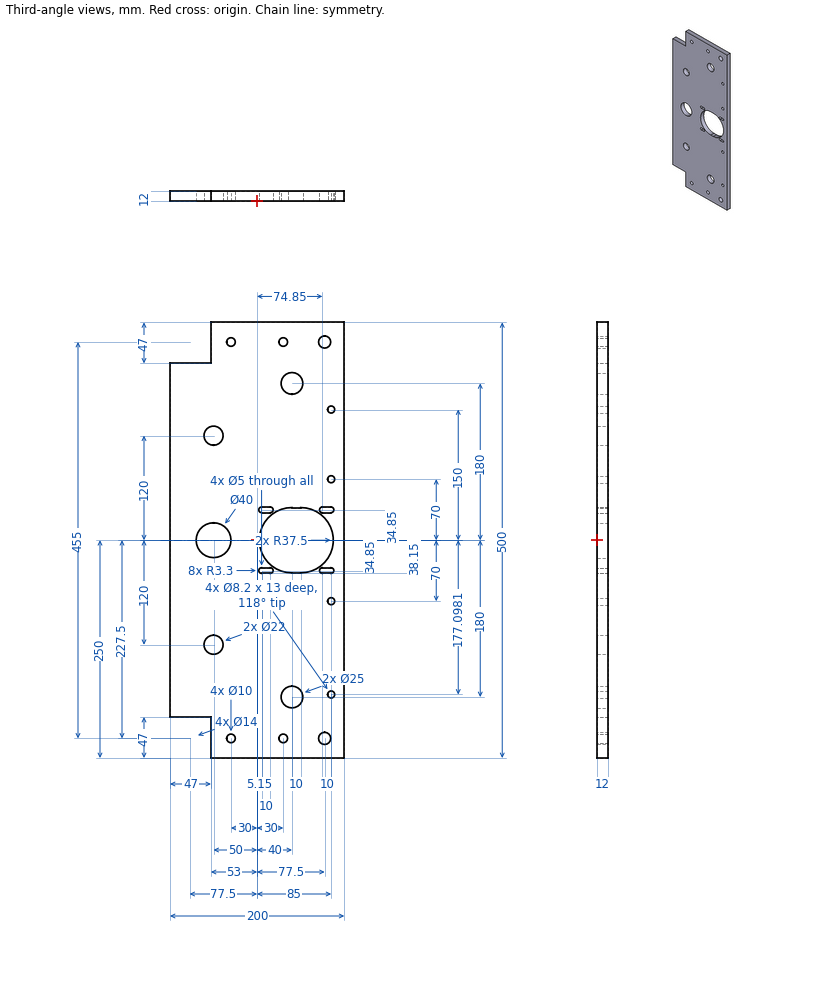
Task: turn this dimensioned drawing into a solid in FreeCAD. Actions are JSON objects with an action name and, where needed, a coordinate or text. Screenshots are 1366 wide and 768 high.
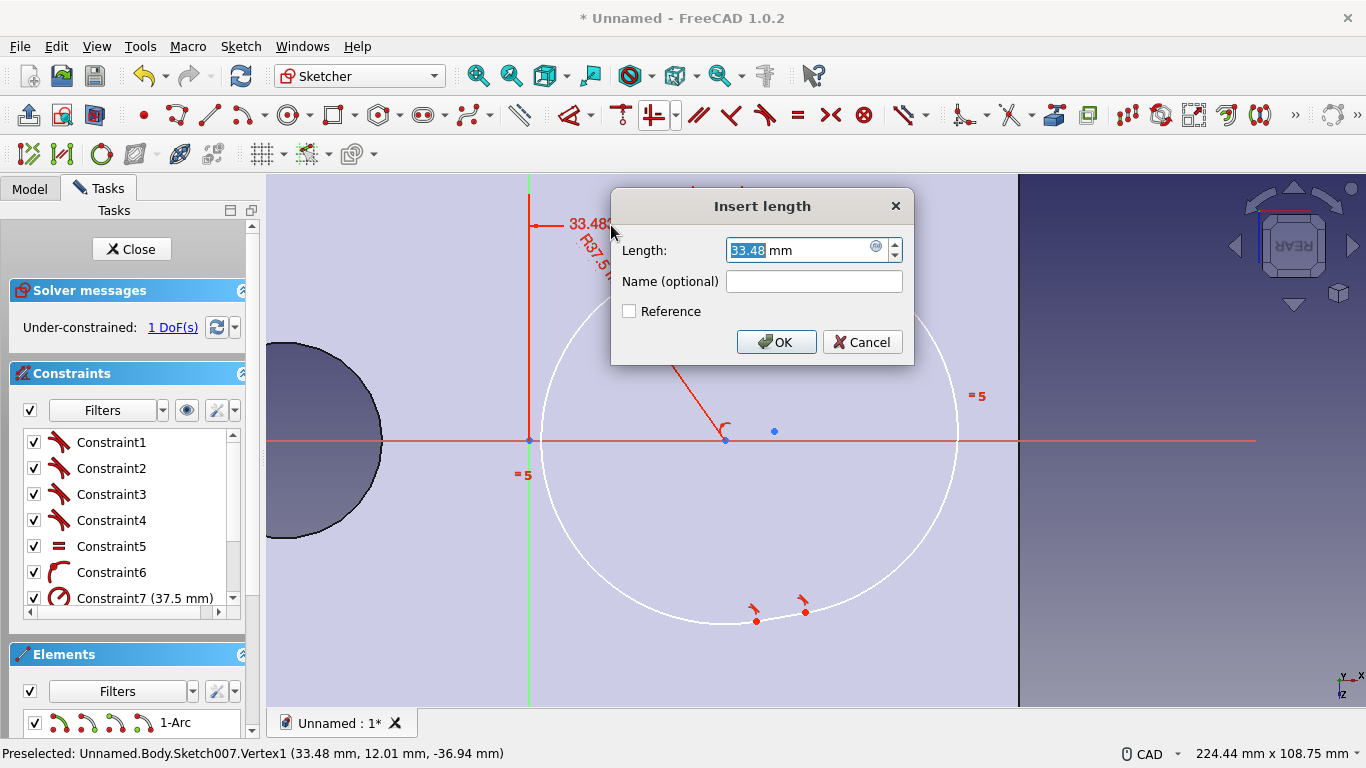
{"action": "type", "text": "40"}
{"action": "key", "text": "Return"}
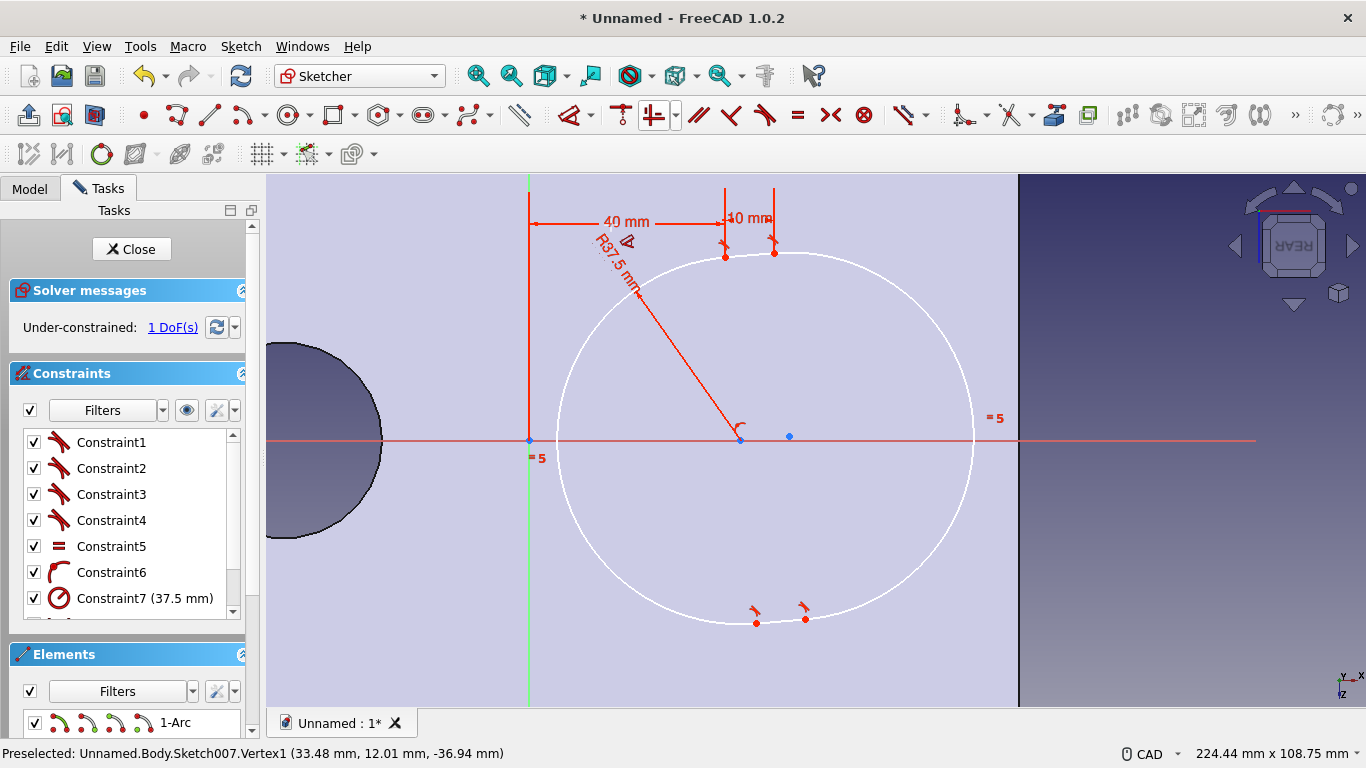
{"action": "left_click", "coordinate": [757, 624]}
{"action": "left_click", "coordinate": [643, 658]}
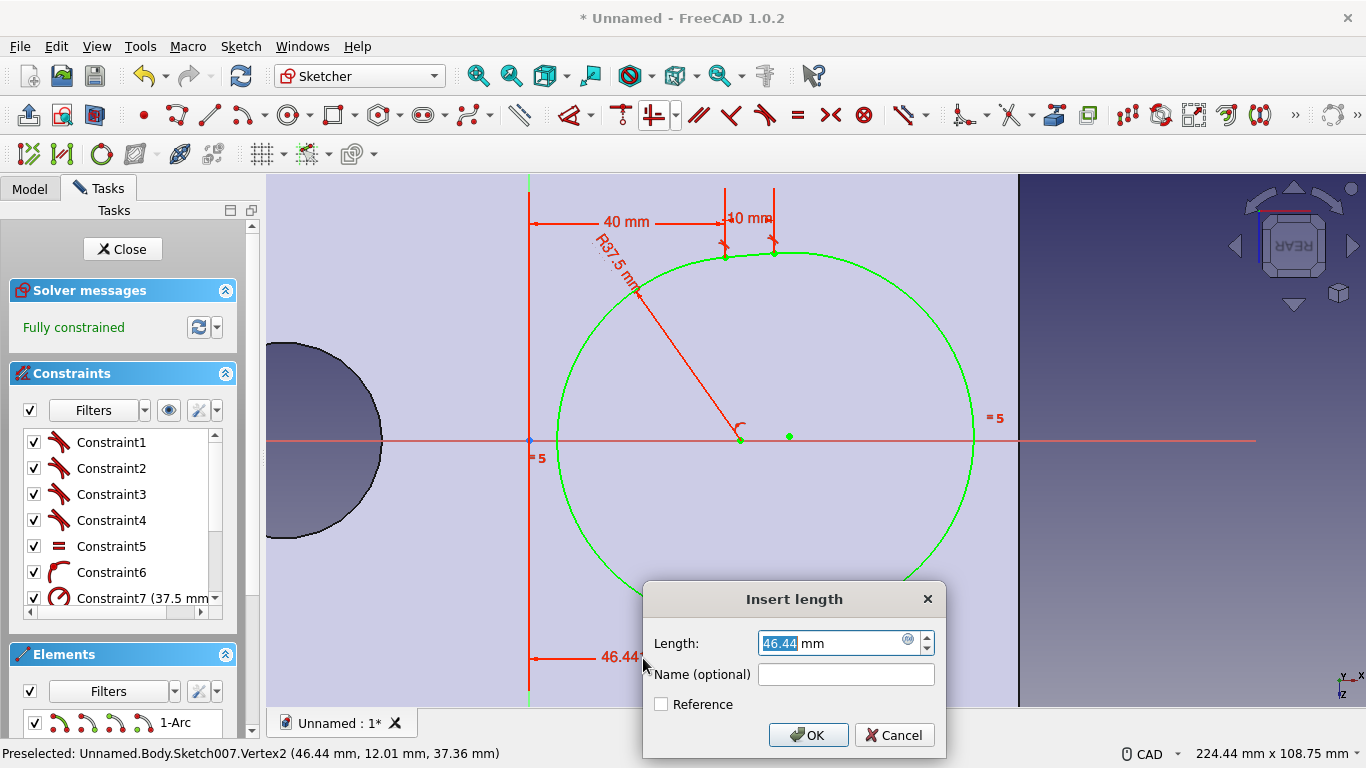
{"action": "type", "text": "40"}
{"action": "key", "text": "Return"}
{"action": "key", "text": "Escape"}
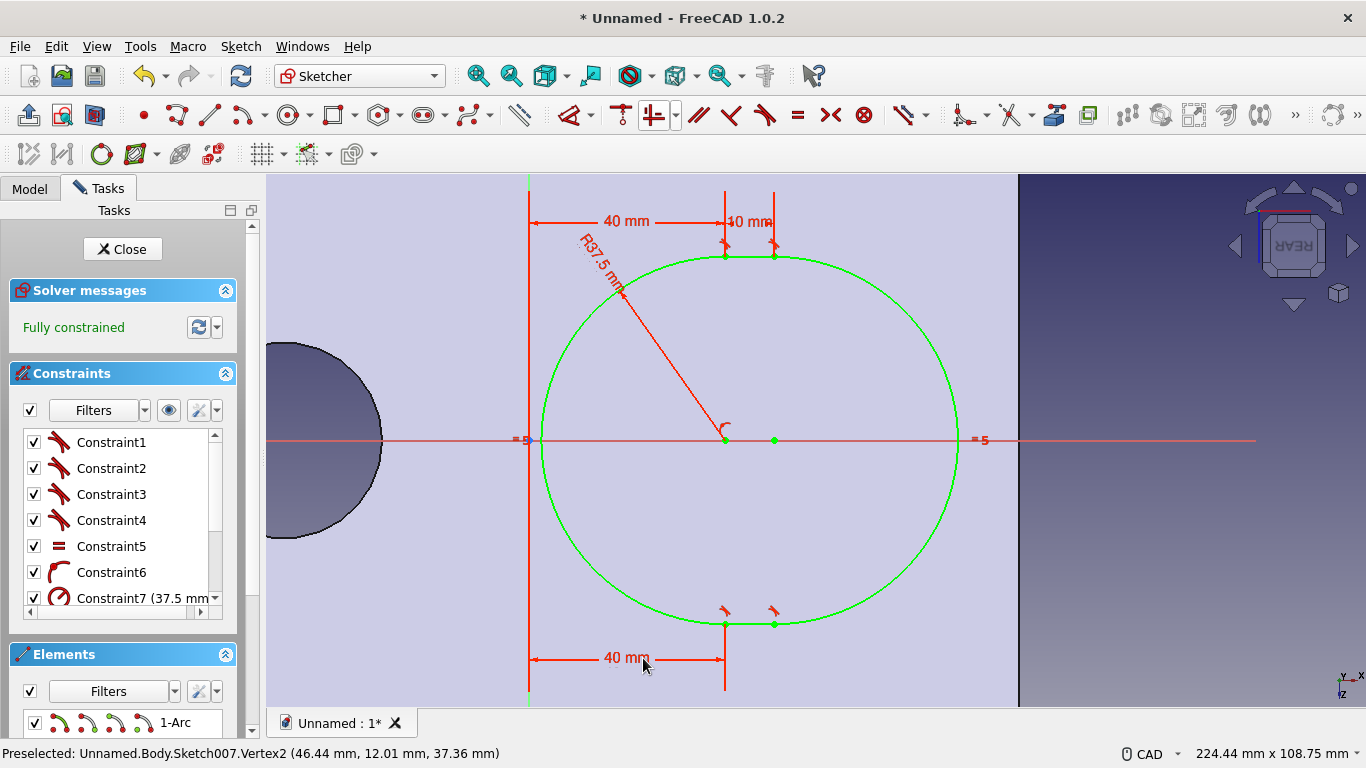
{"action": "left_click", "coordinate": [123, 249]}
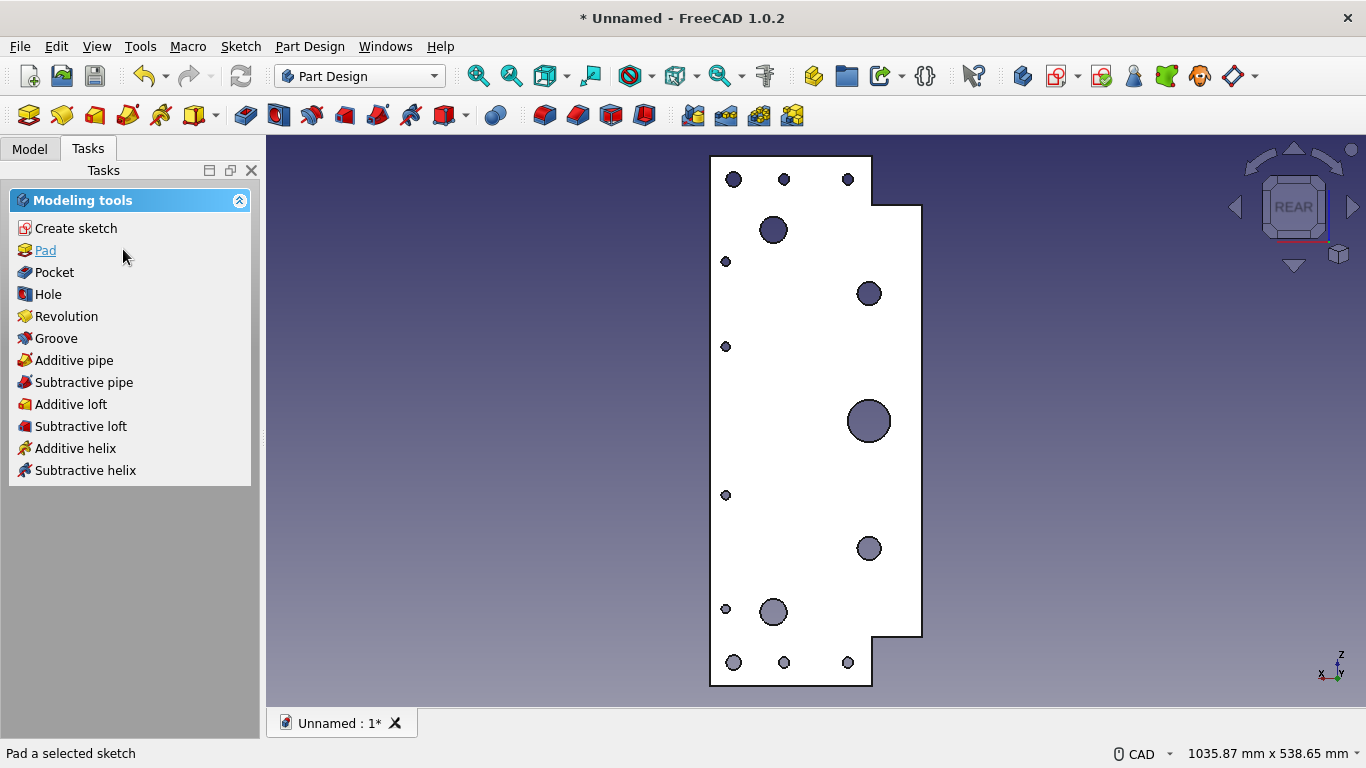
{"action": "left_click", "coordinate": [246, 116]}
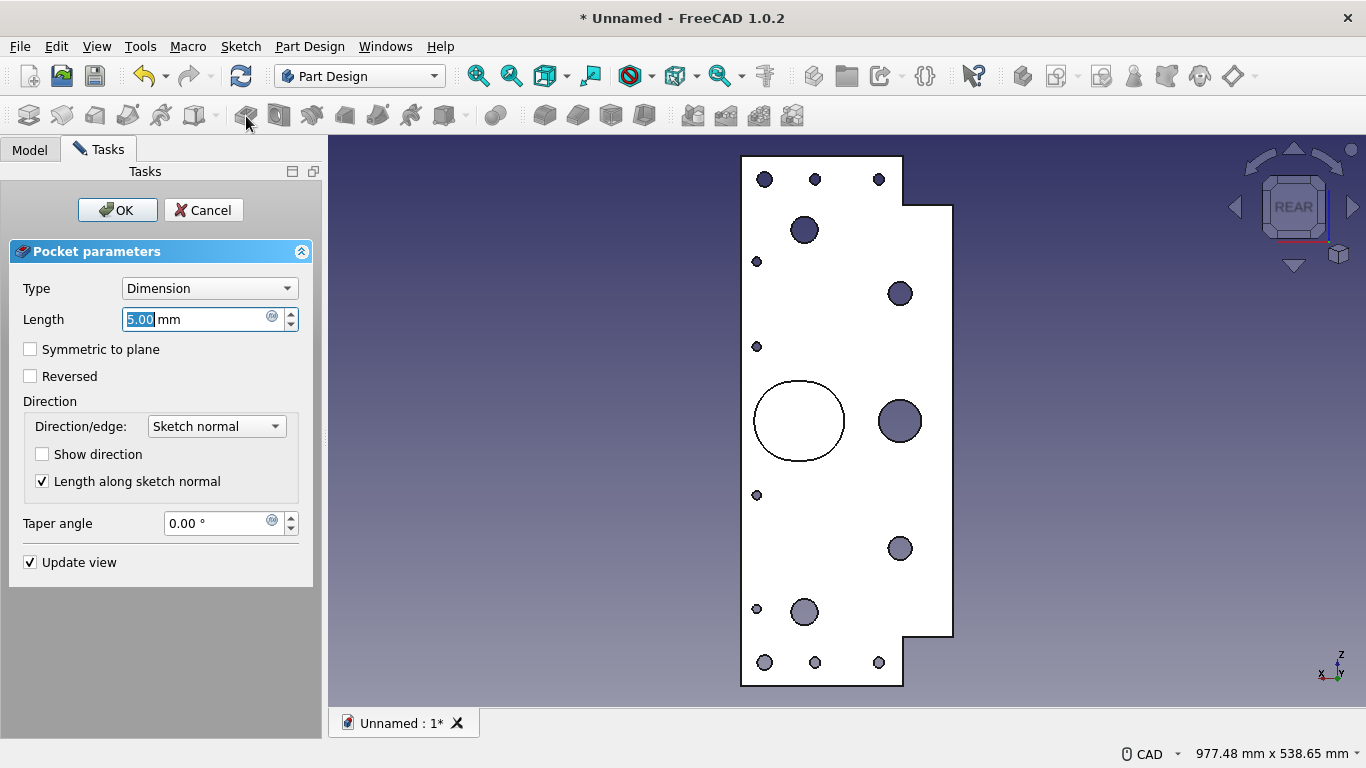
{"action": "left_click", "coordinate": [210, 288]}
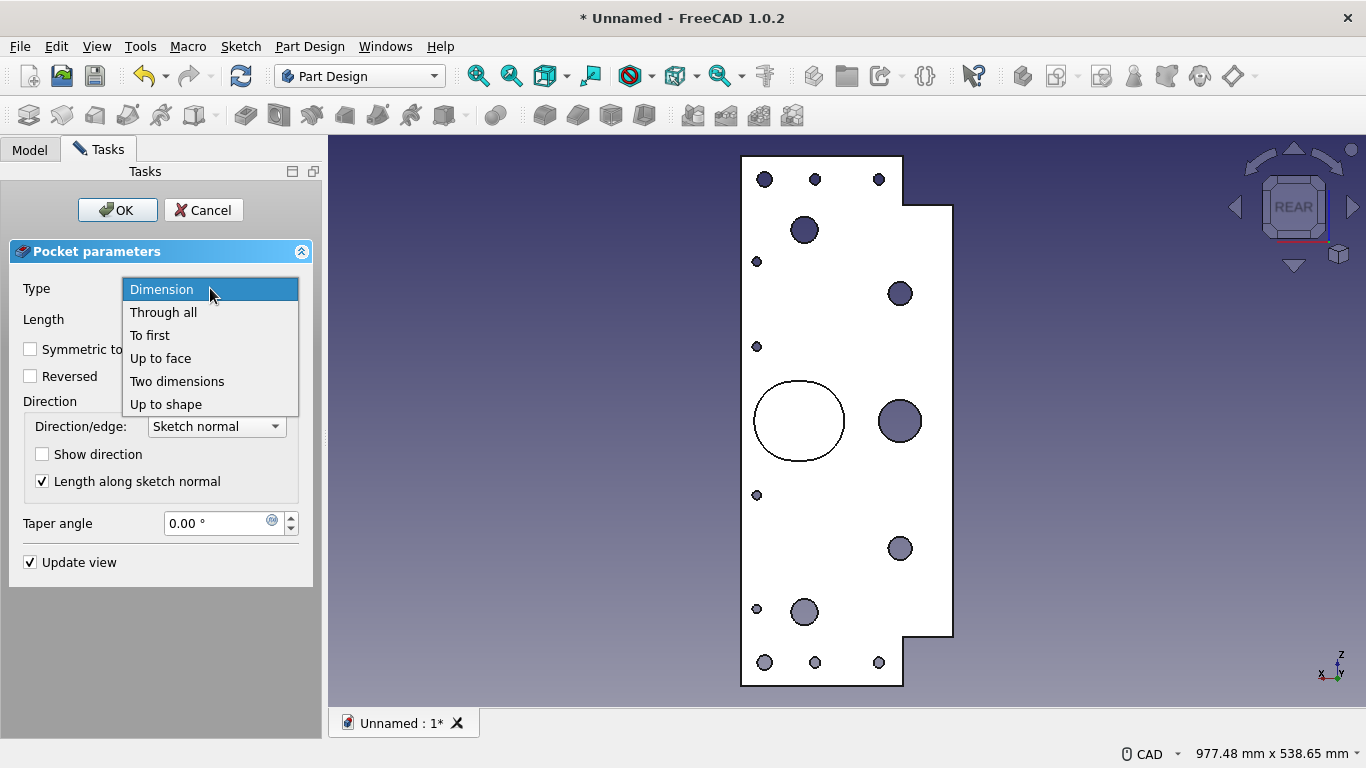
{"action": "left_click", "coordinate": [208, 312]}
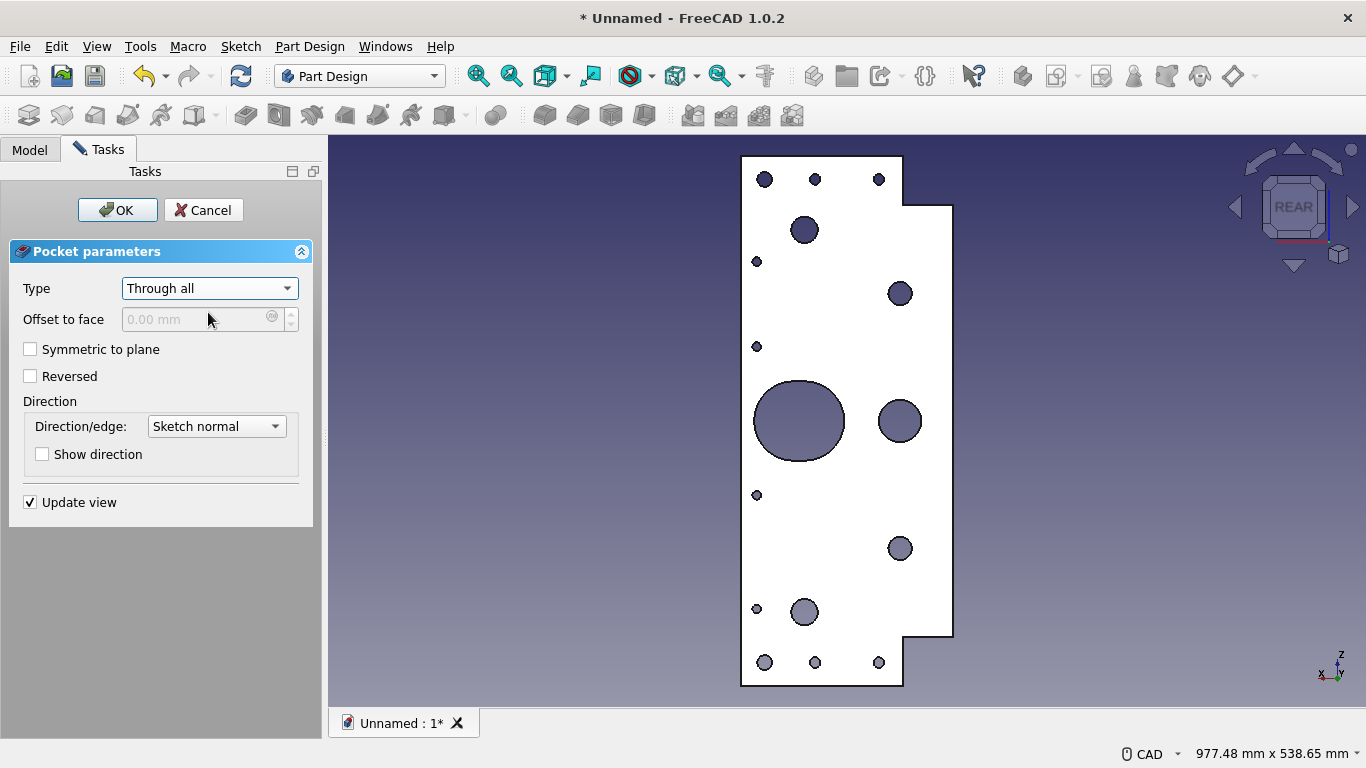
{"action": "left_click", "coordinate": [118, 210]}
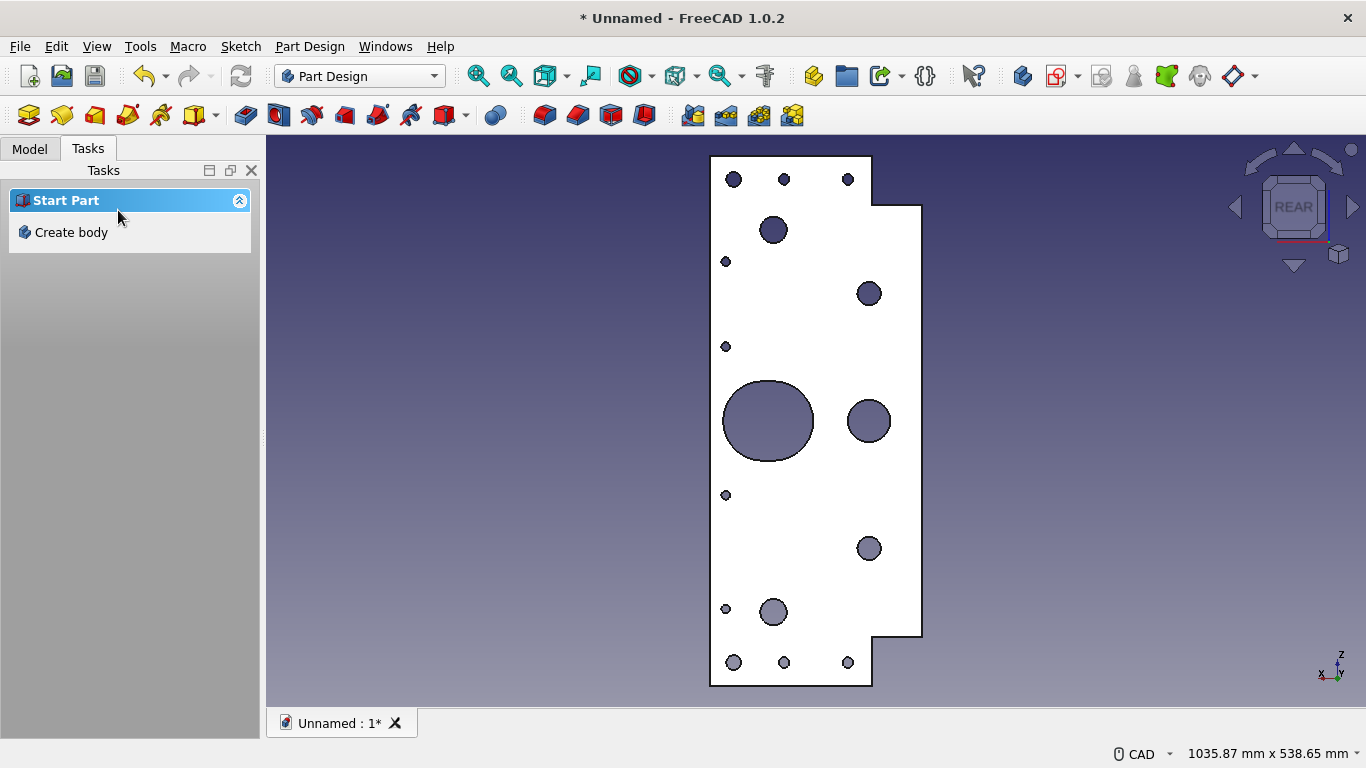
{"action": "left_click", "coordinate": [816, 344]}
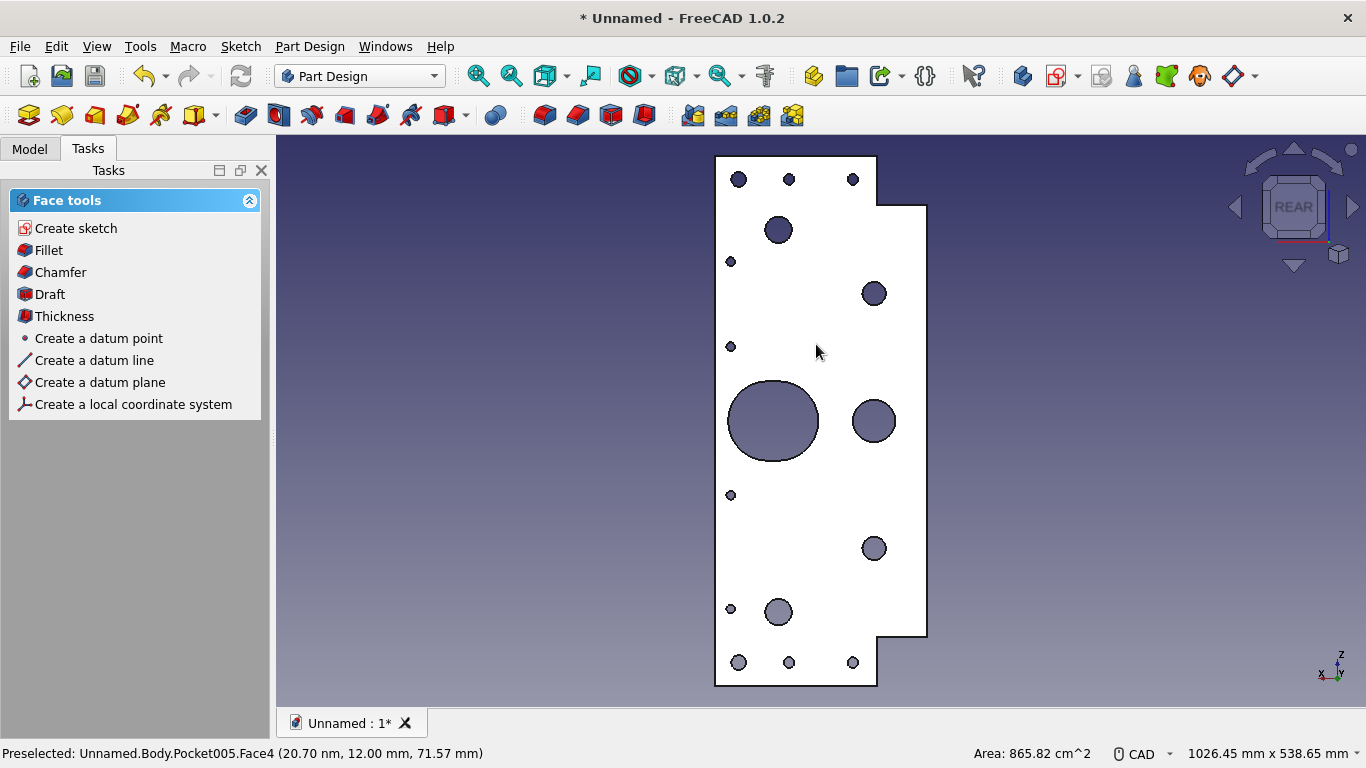
{"action": "left_click", "coordinate": [1056, 76]}